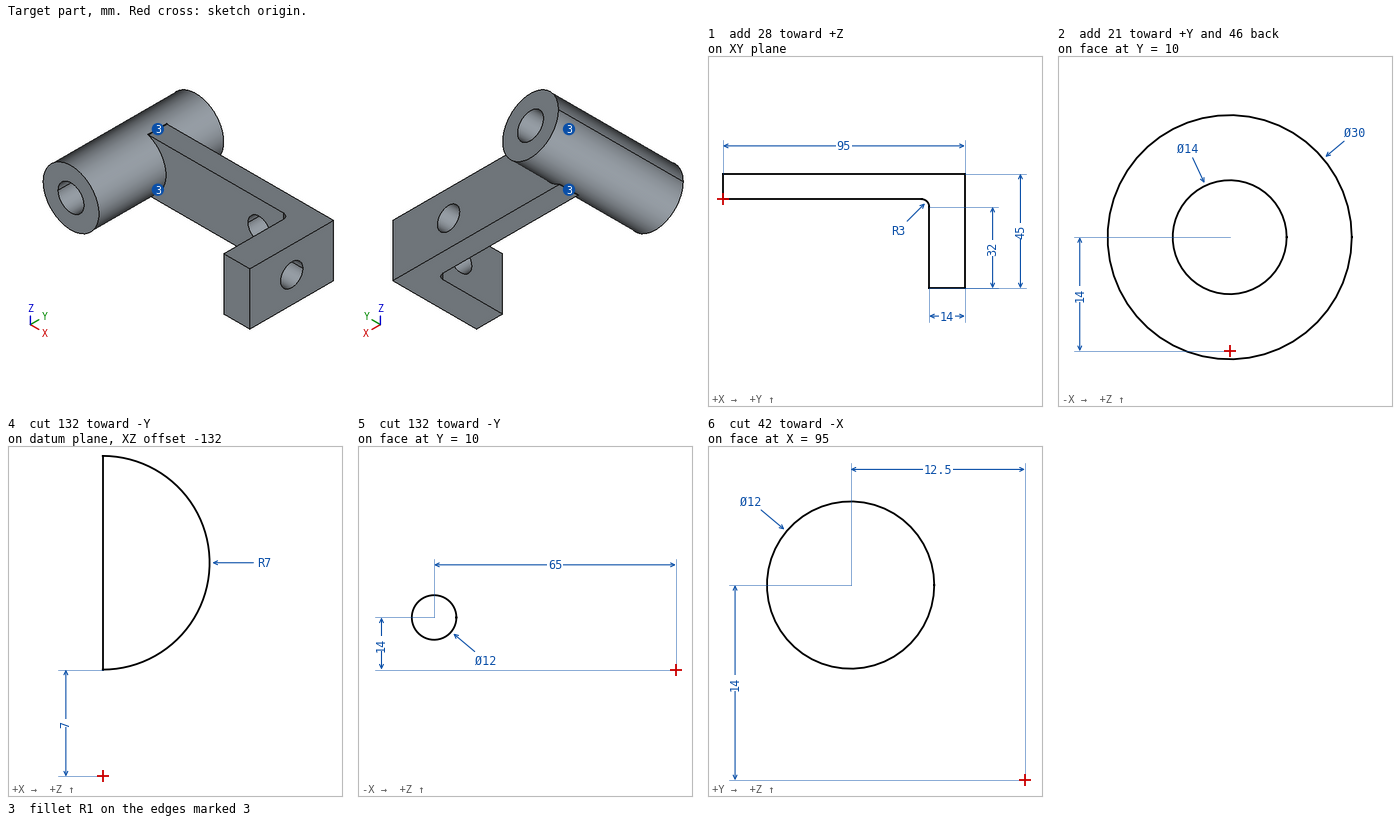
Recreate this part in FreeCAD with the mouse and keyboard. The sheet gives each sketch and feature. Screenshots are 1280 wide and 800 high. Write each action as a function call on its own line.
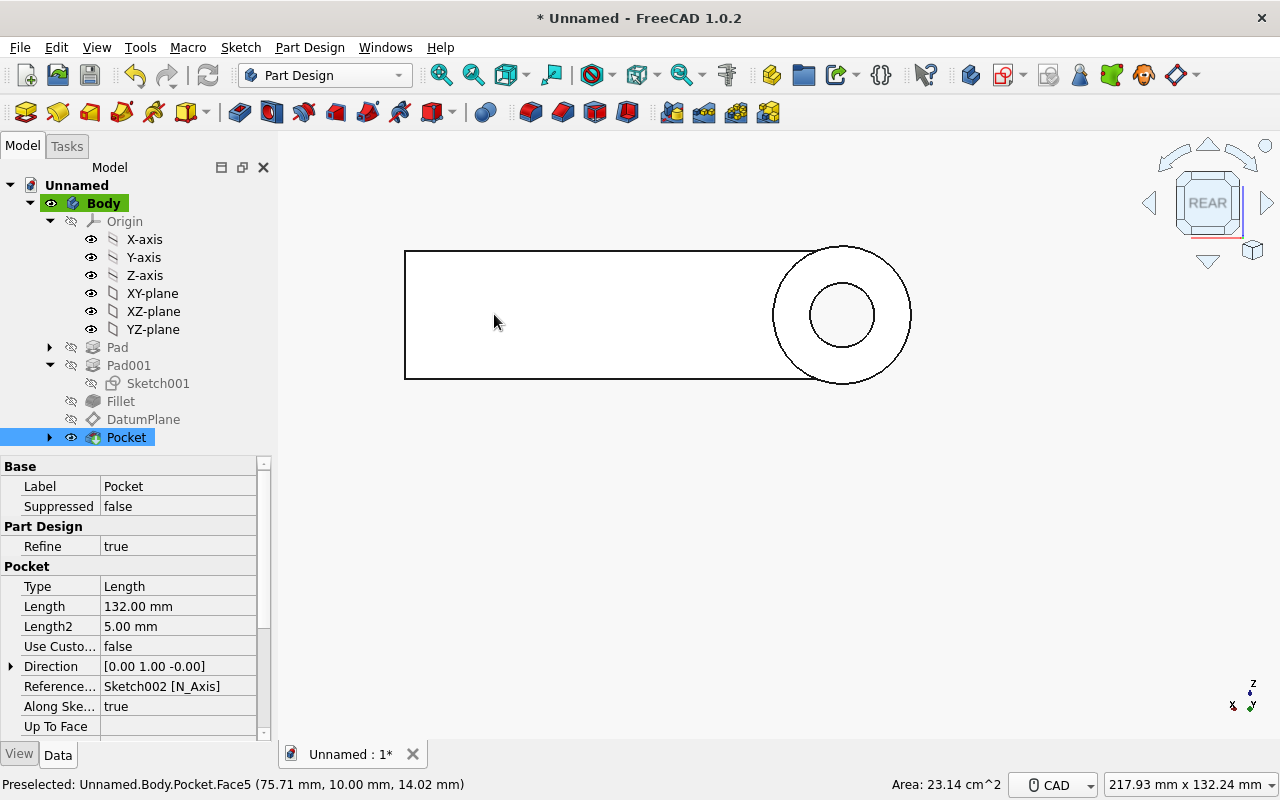
click(1004, 76)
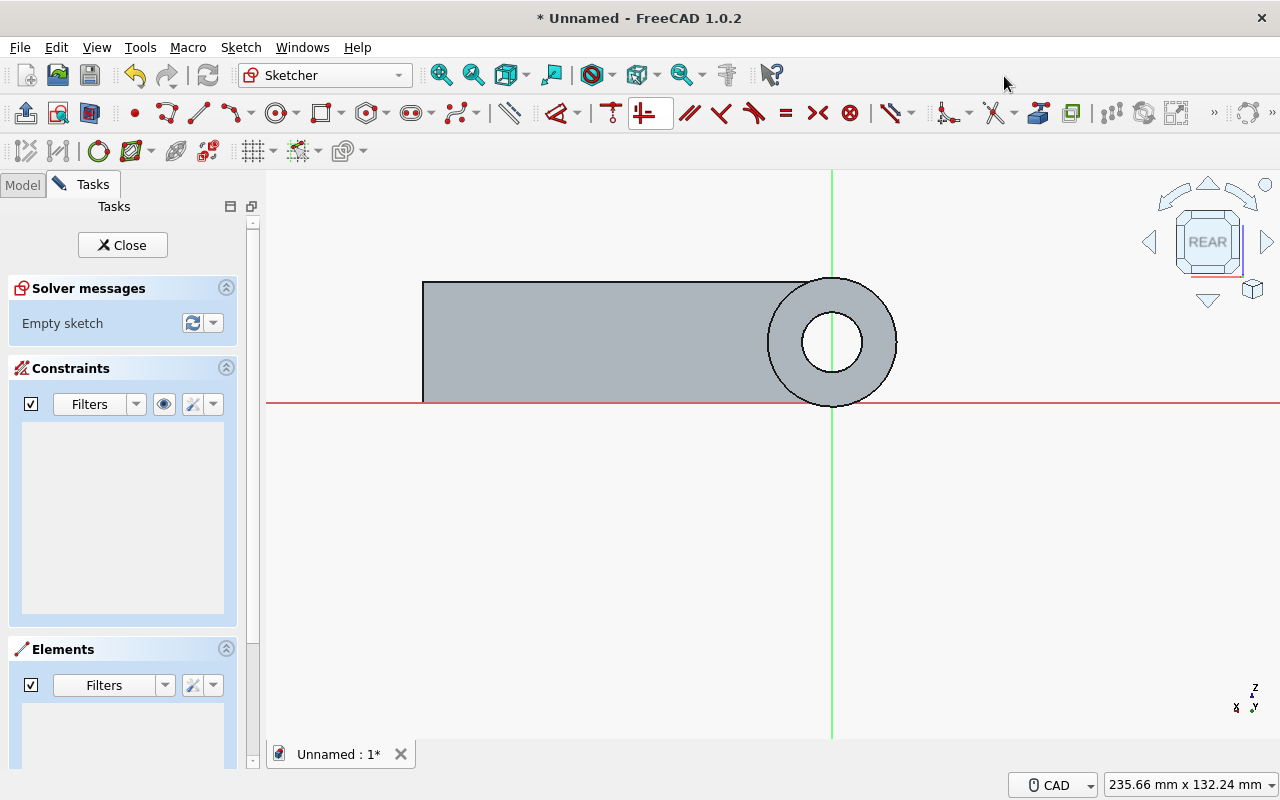
click(90, 114)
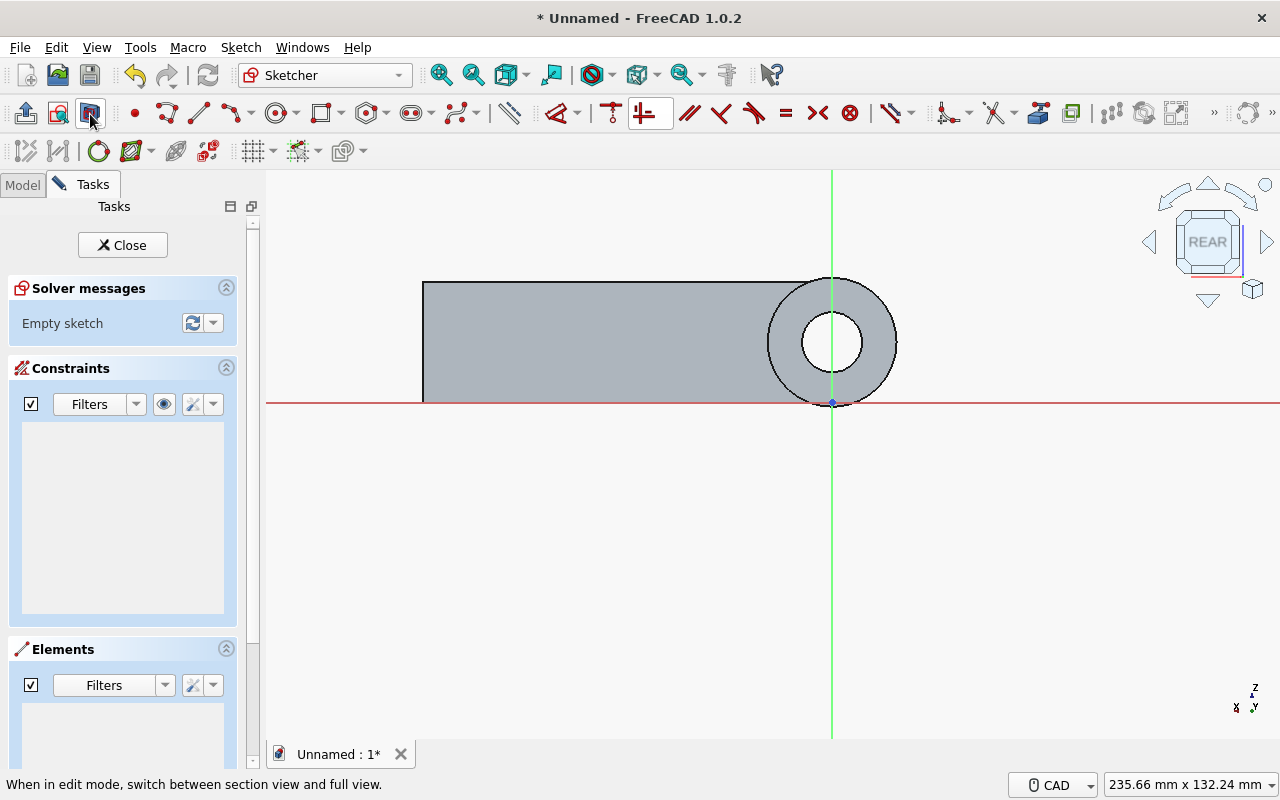
scroll(529, 325, up, 10)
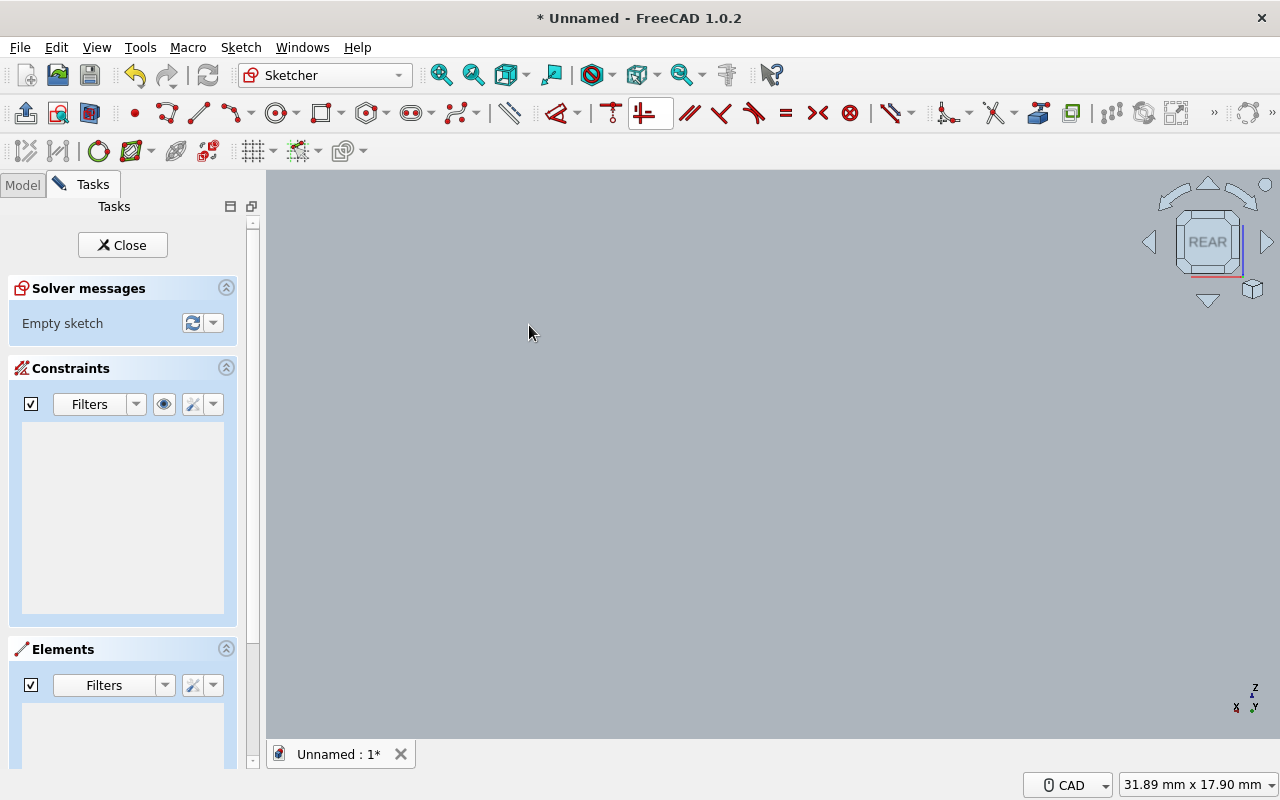
click(276, 114)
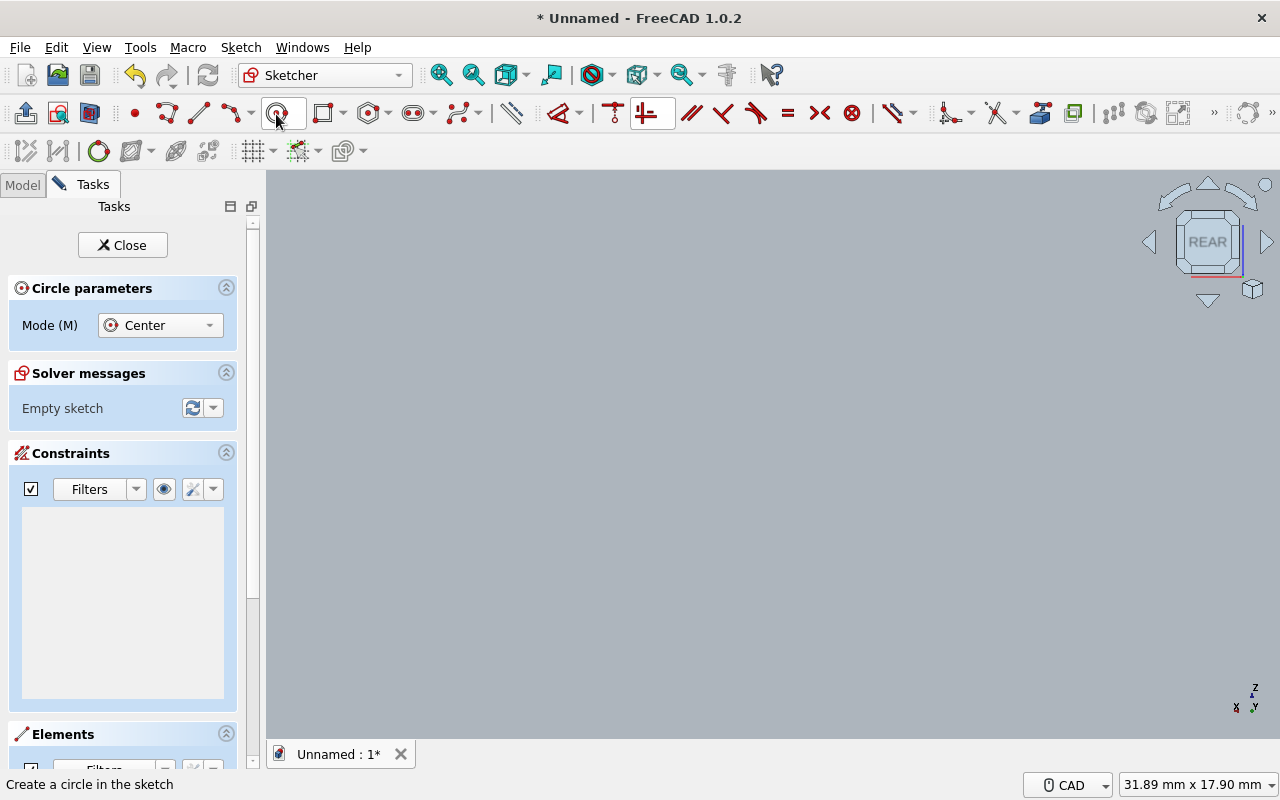
click(700, 451)
move(835, 316)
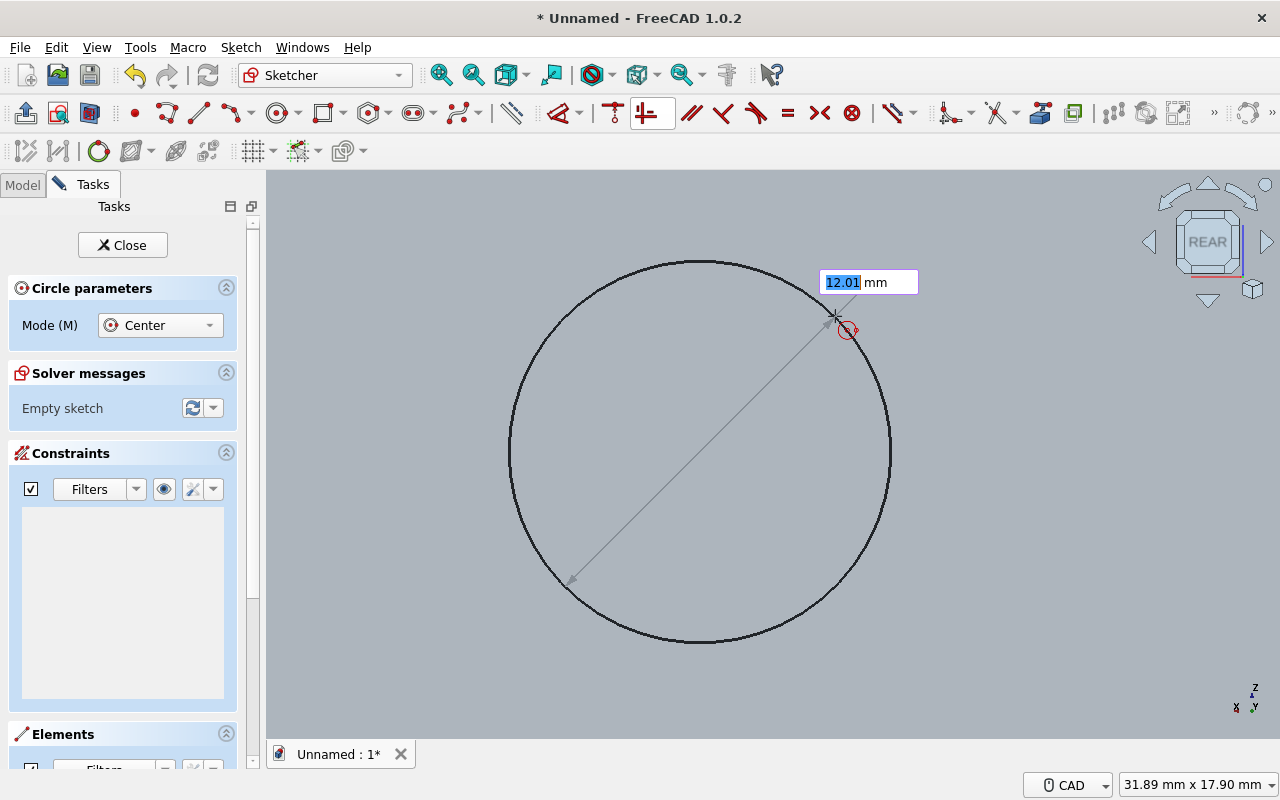
text(12)
key(Return)
key(Escape)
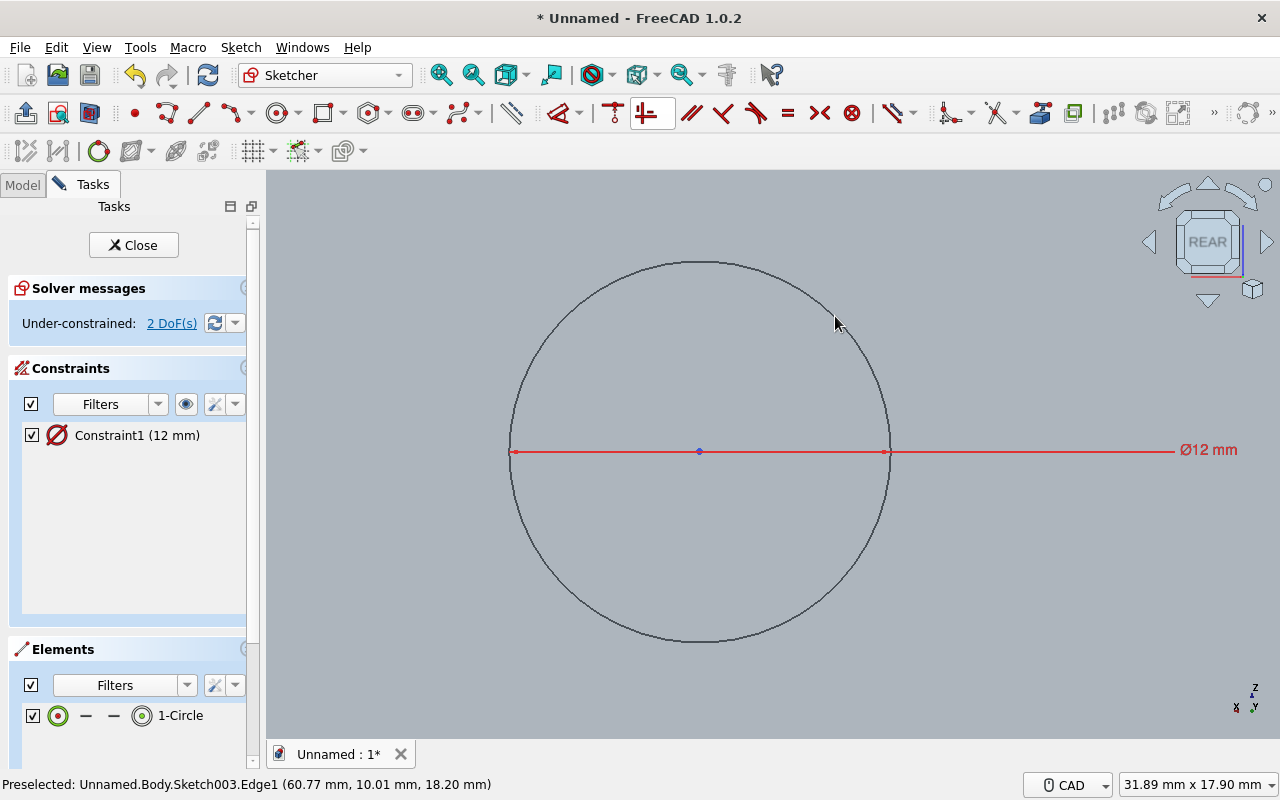
click(558, 114)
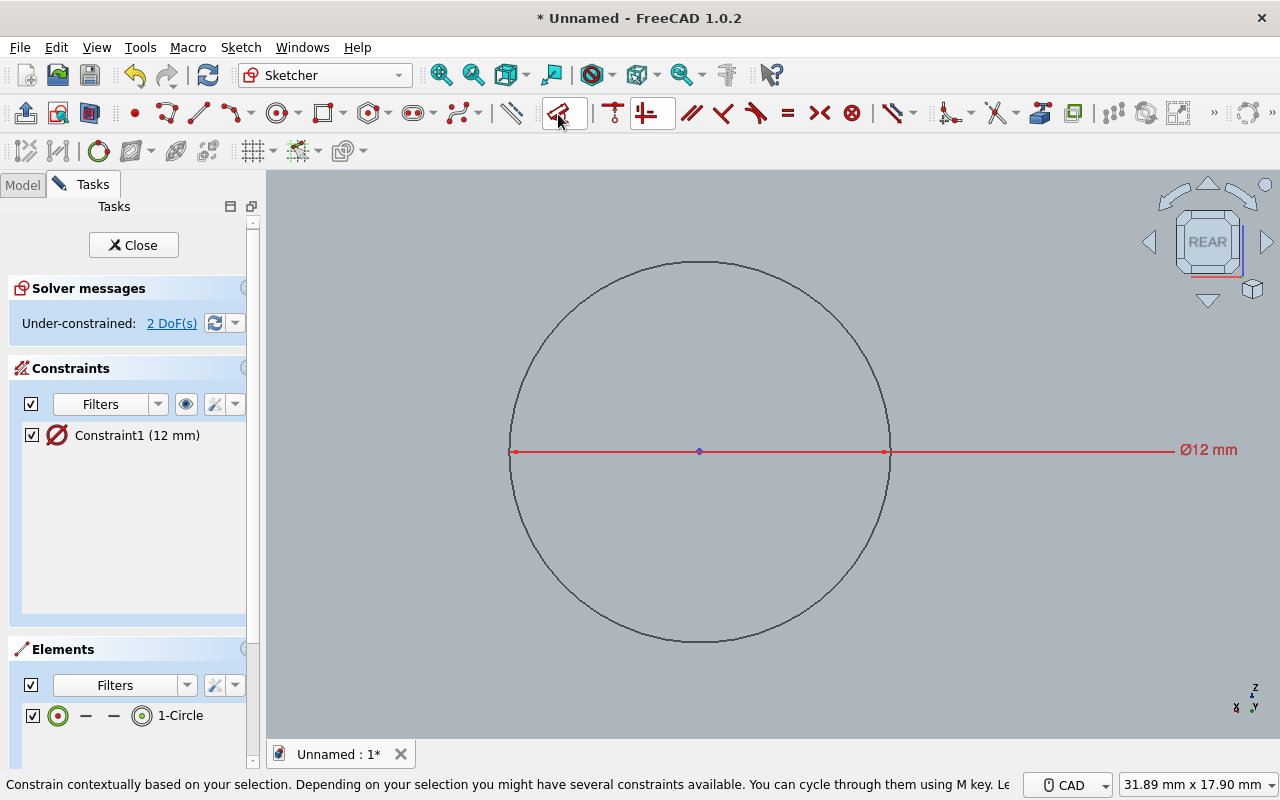
click(700, 452)
click(908, 418)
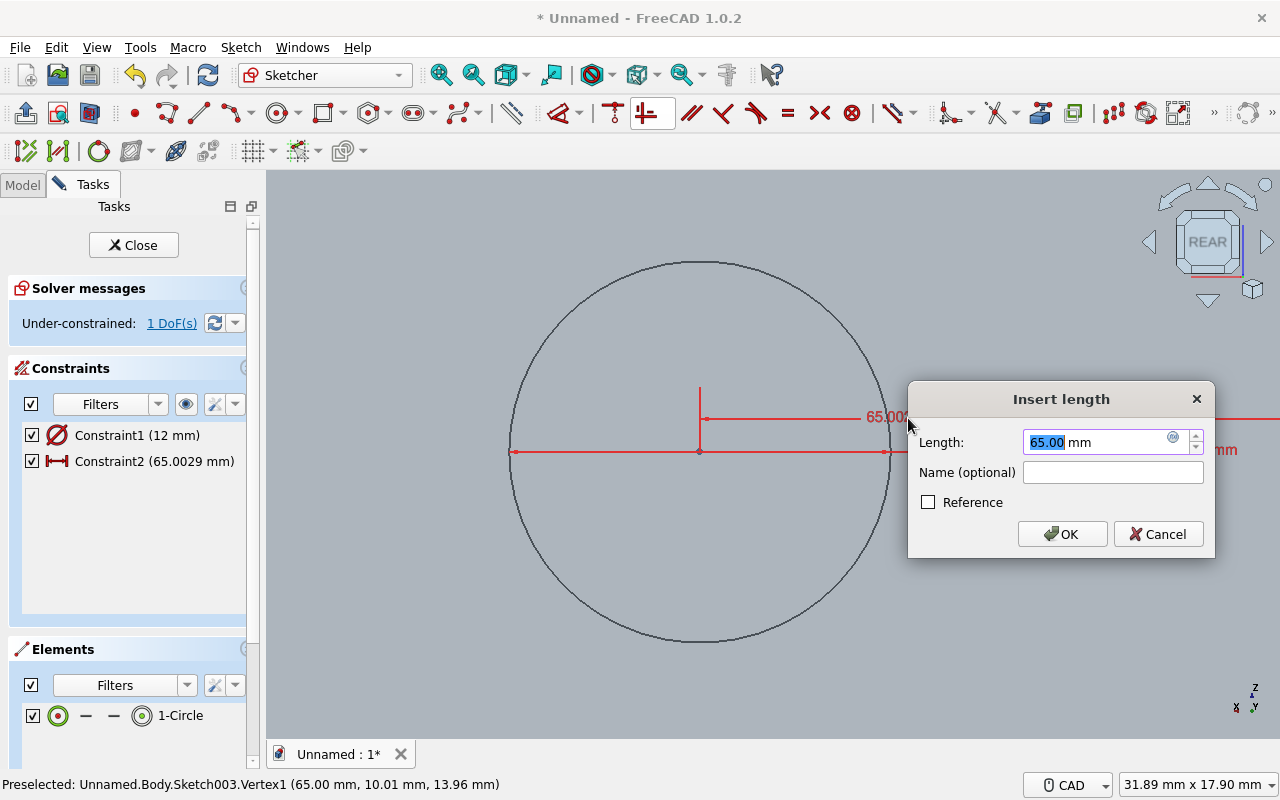
text(65)
key(Return)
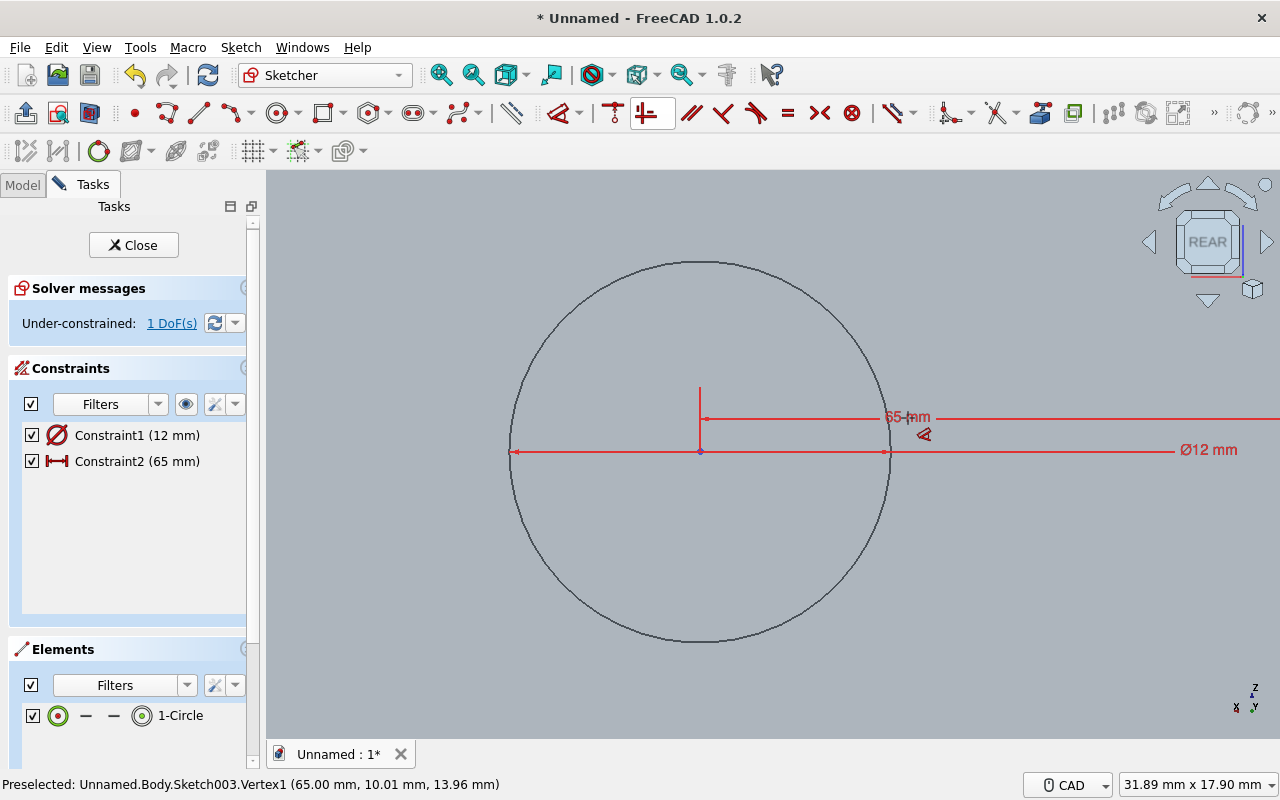
click(700, 452)
click(666, 581)